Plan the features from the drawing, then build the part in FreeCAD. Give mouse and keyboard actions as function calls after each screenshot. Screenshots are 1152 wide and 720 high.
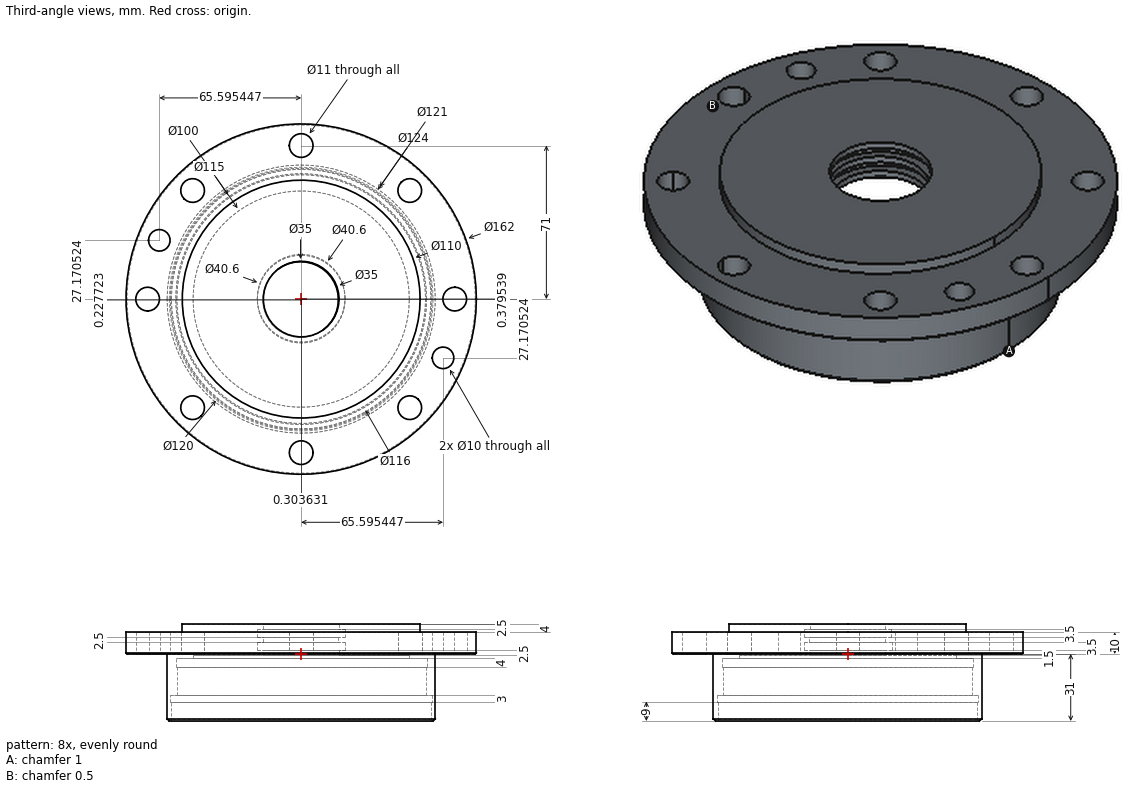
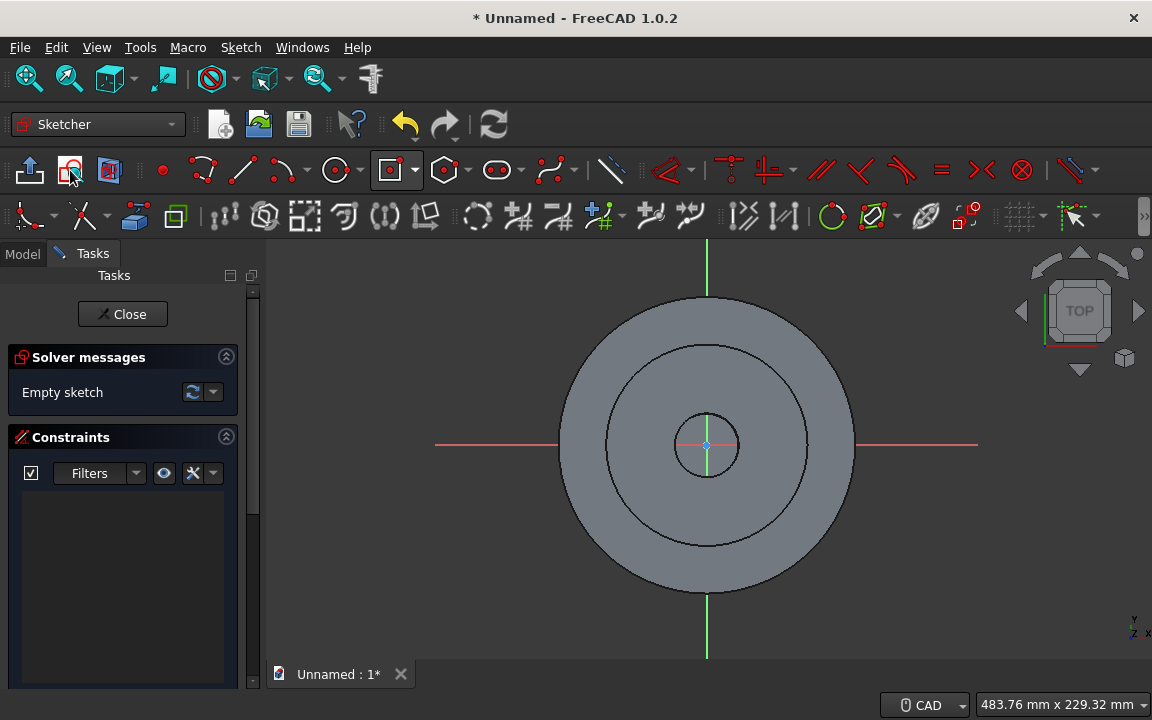
scroll(842, 438, up, 2)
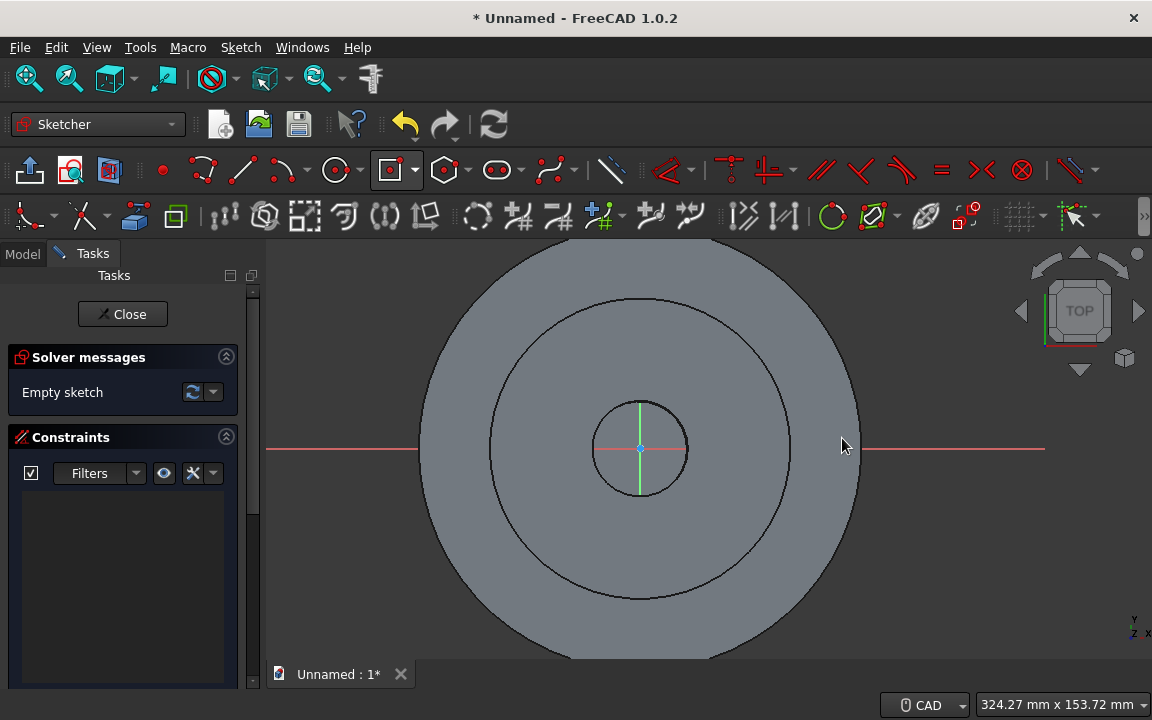
click(336, 170)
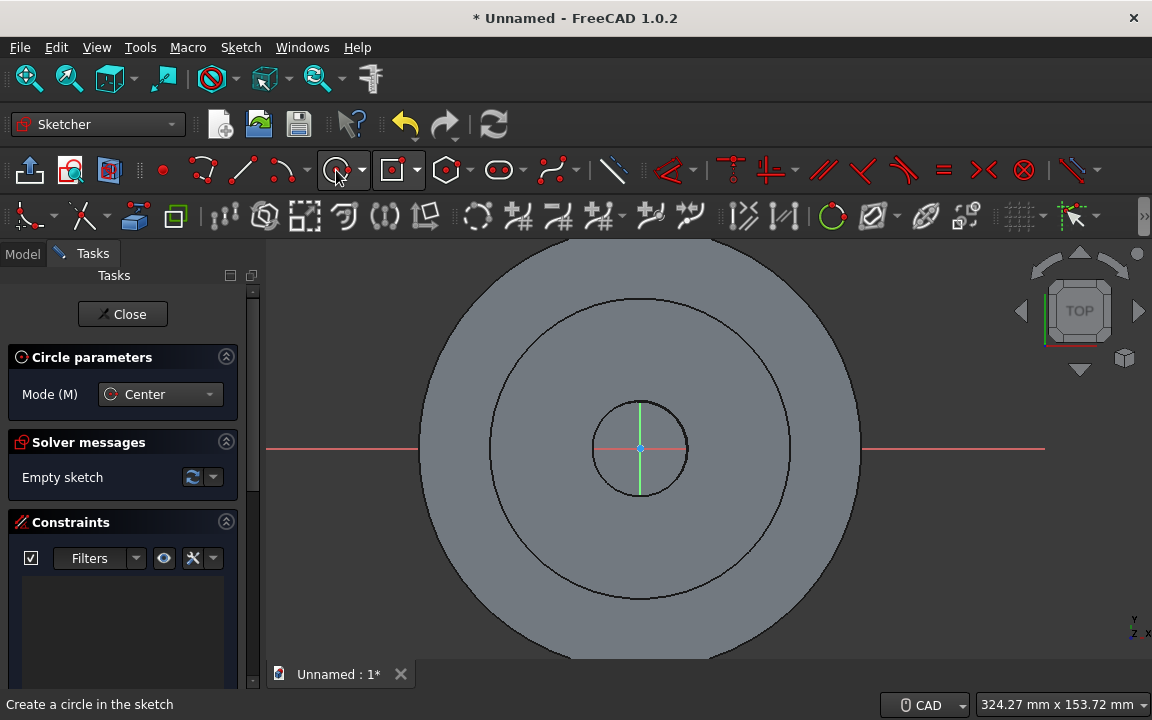
click(640, 449)
click(737, 352)
key(Escape)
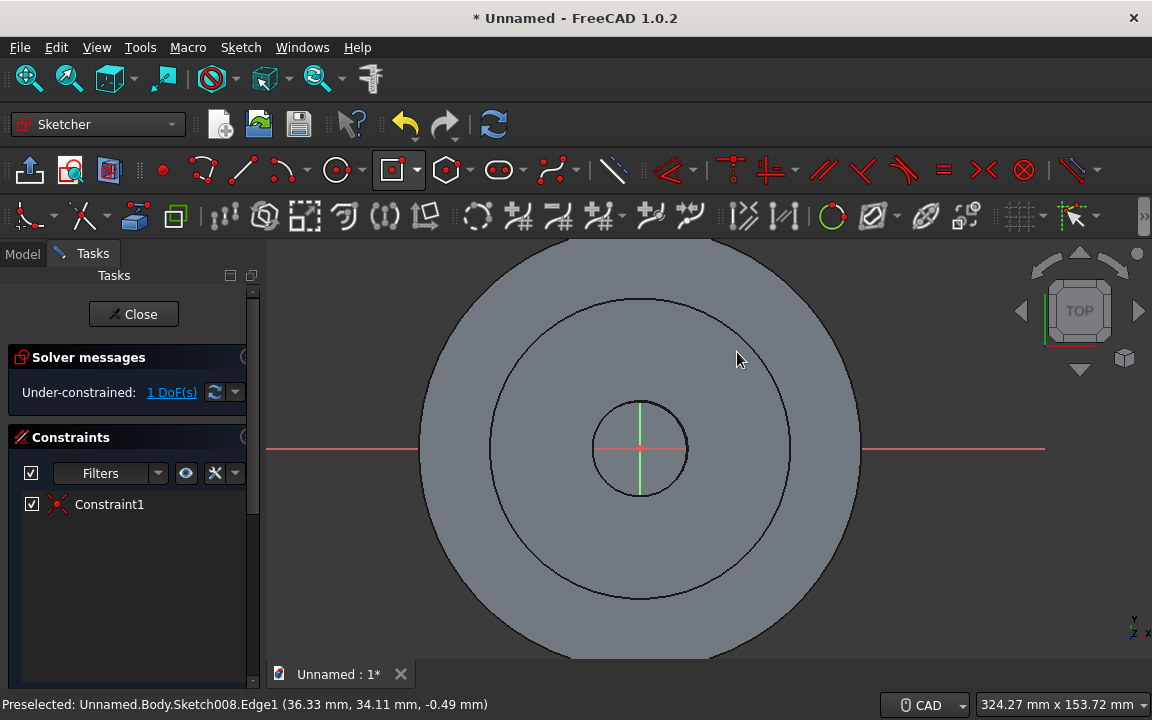
click(668, 170)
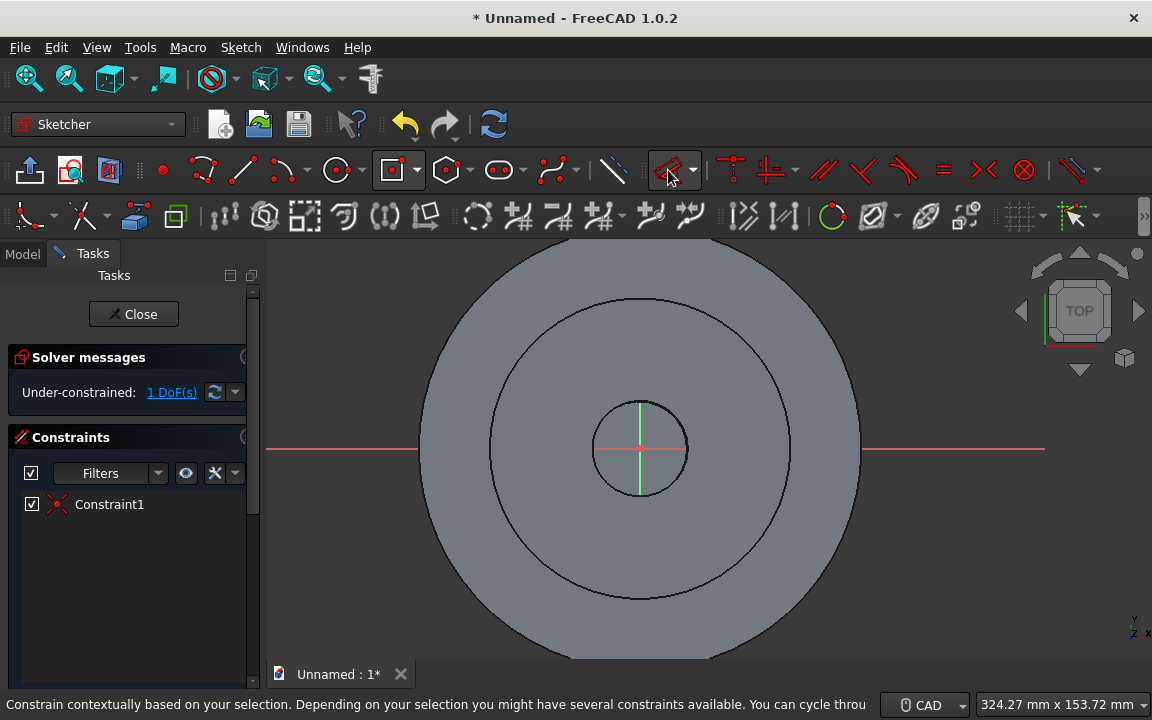
click(736, 352)
click(759, 329)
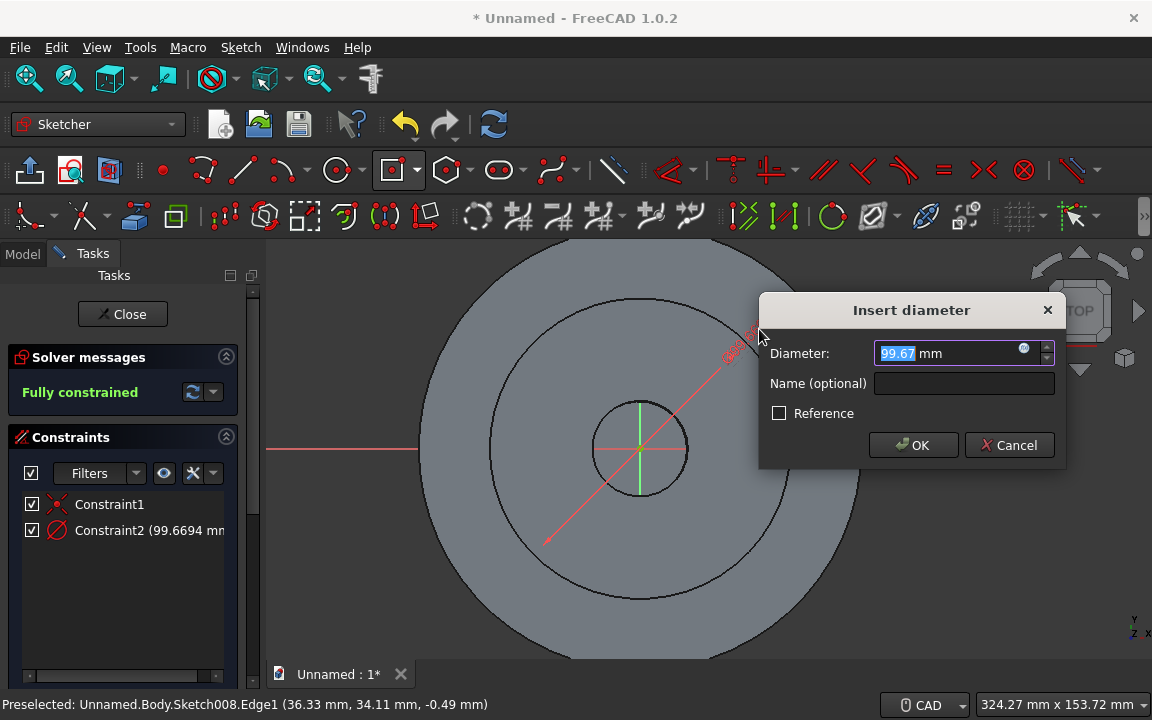
text(100)
key(Return)
key(Escape)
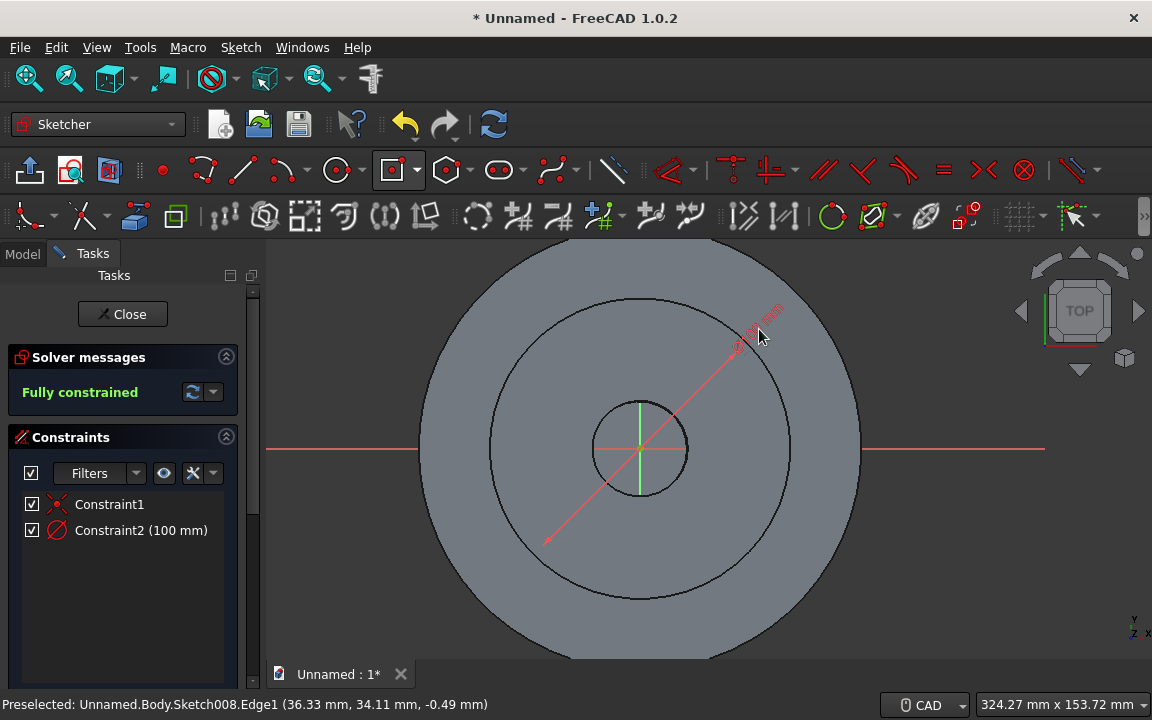
click(123, 314)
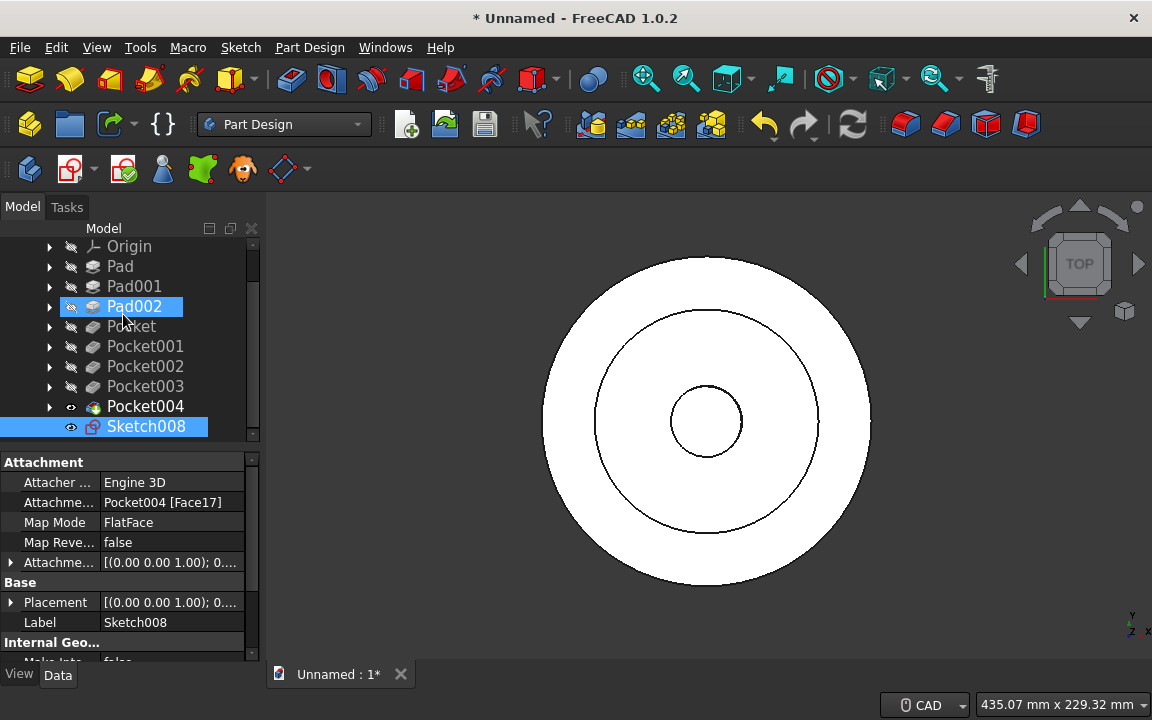
click(292, 80)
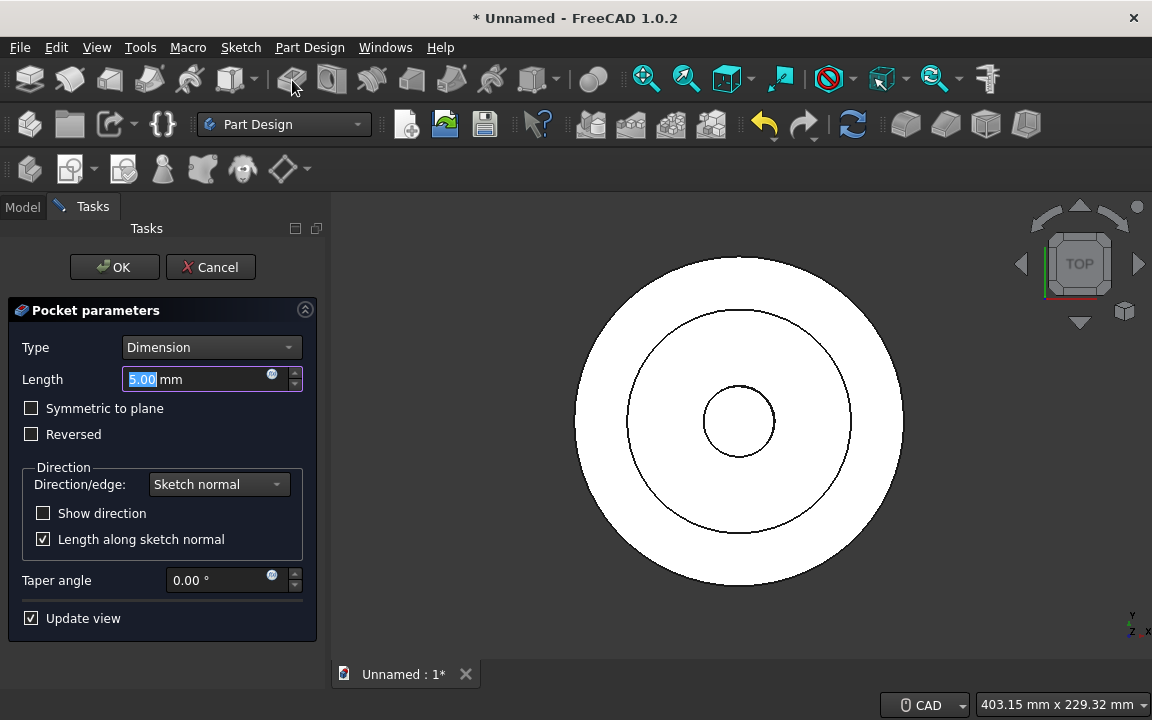
text(1.5)
key(Tab)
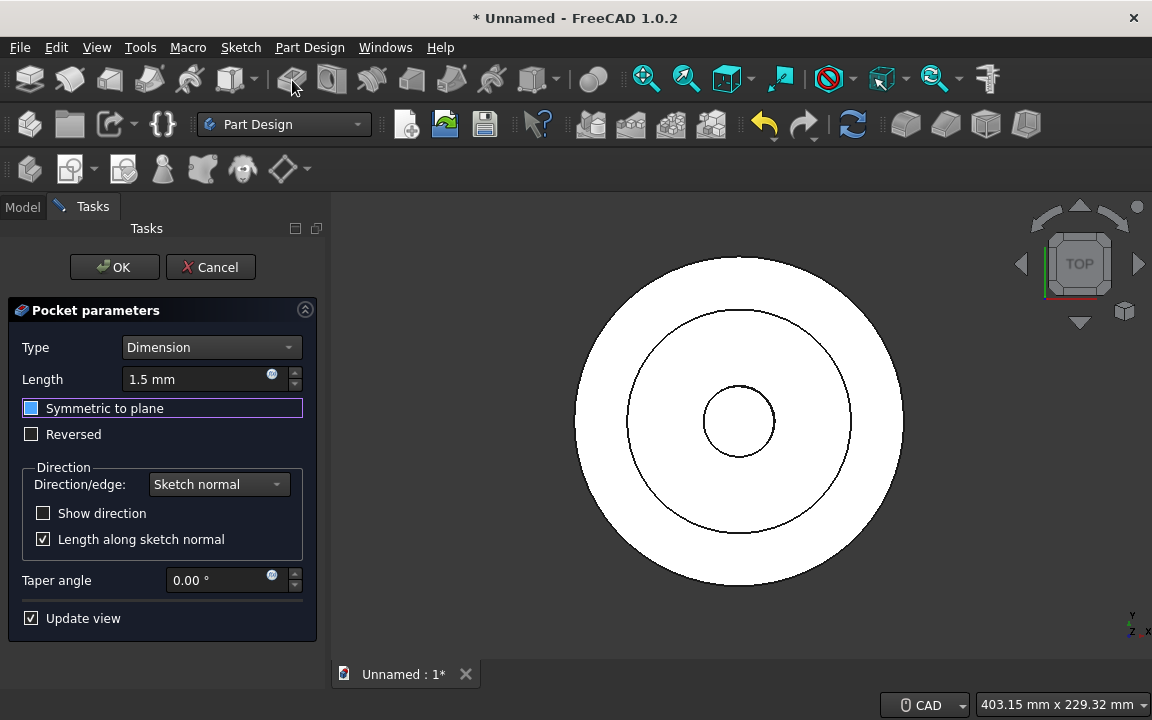
click(115, 267)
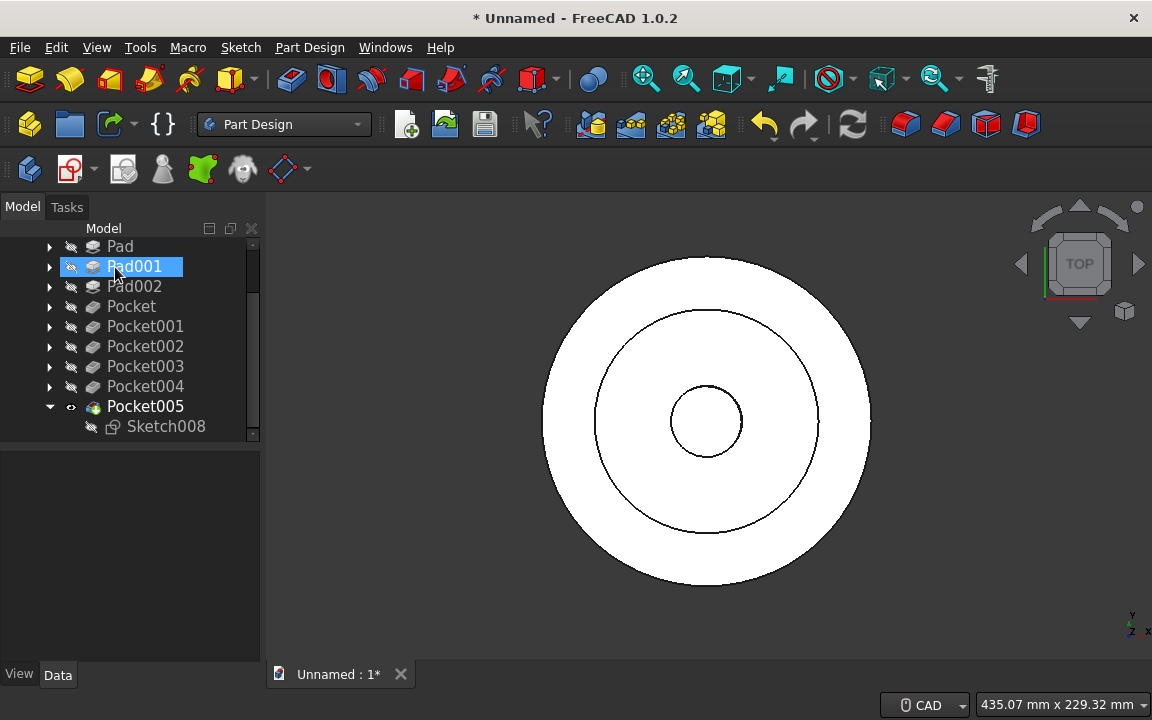
click(848, 420)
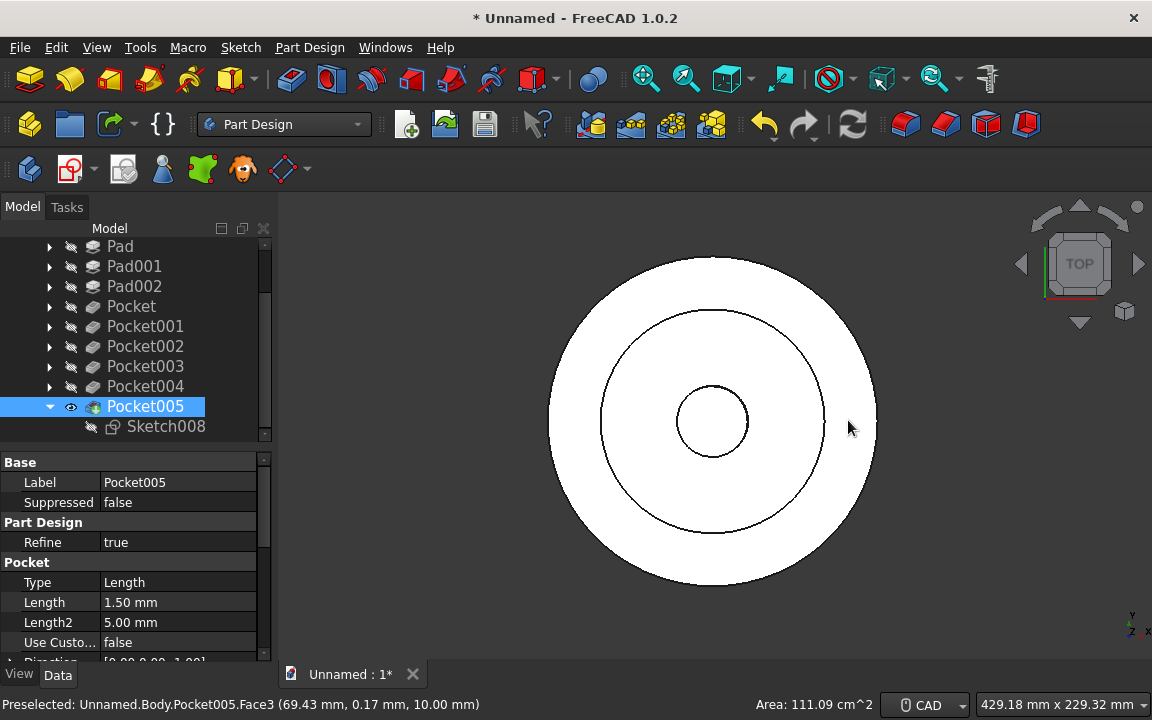
click(70, 170)